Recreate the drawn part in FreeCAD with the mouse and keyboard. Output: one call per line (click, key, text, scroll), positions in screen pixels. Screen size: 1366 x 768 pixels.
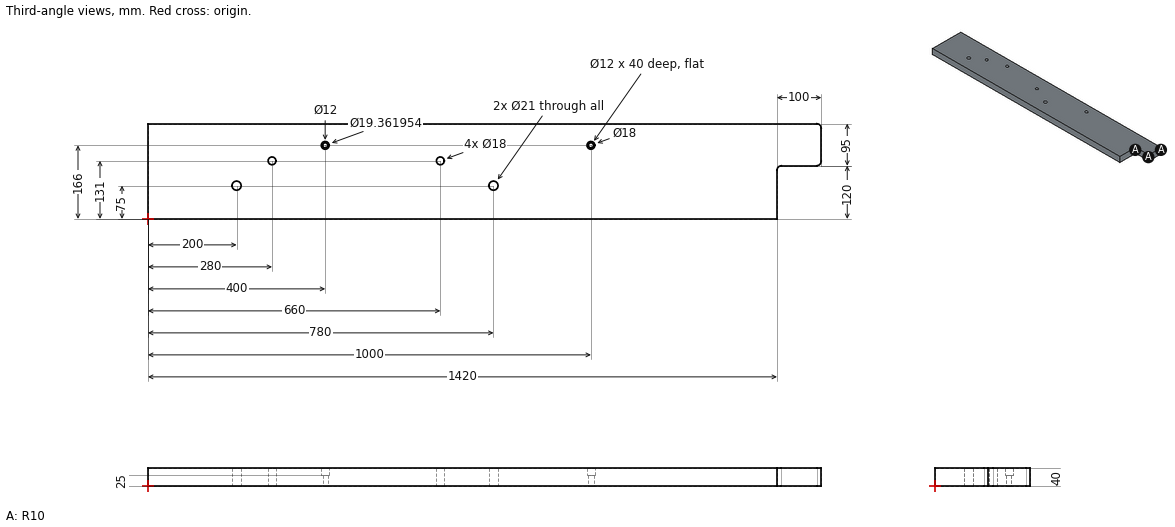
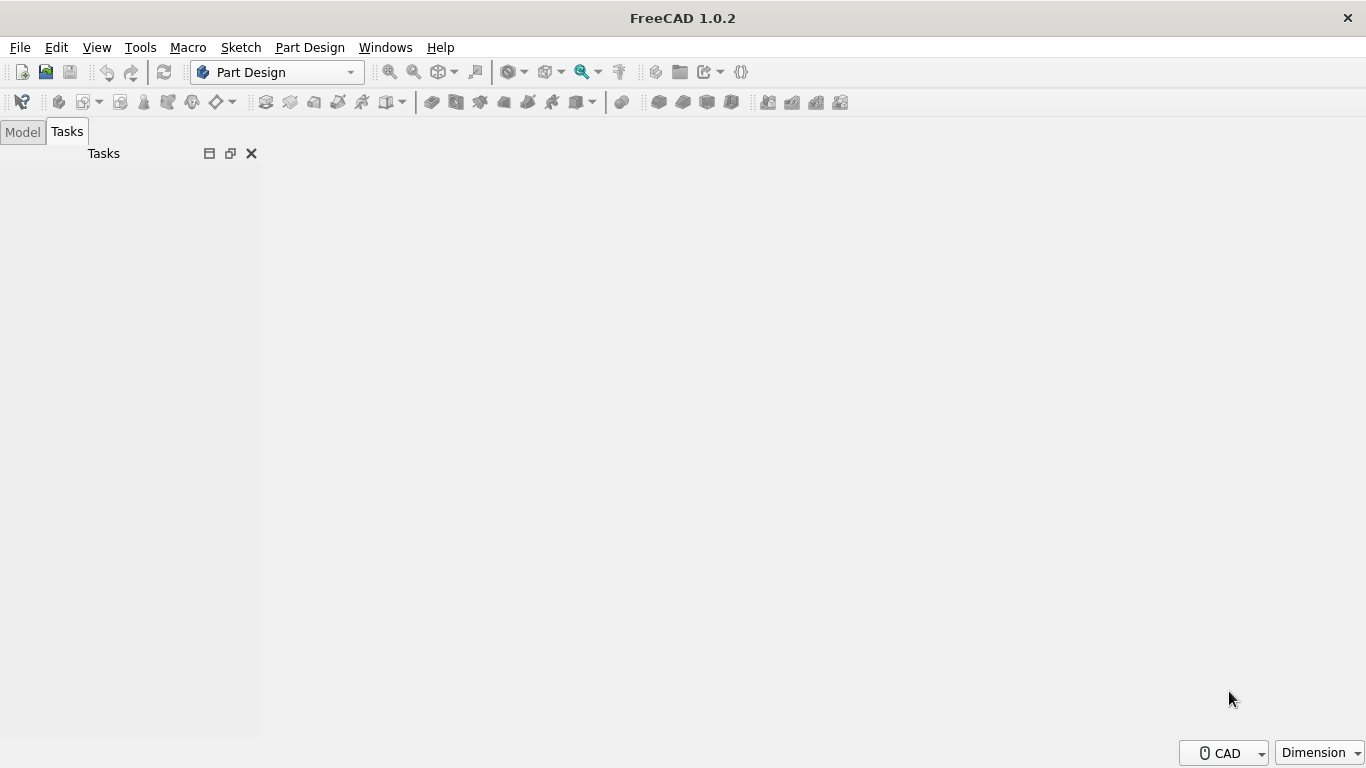
key(ctrl+n)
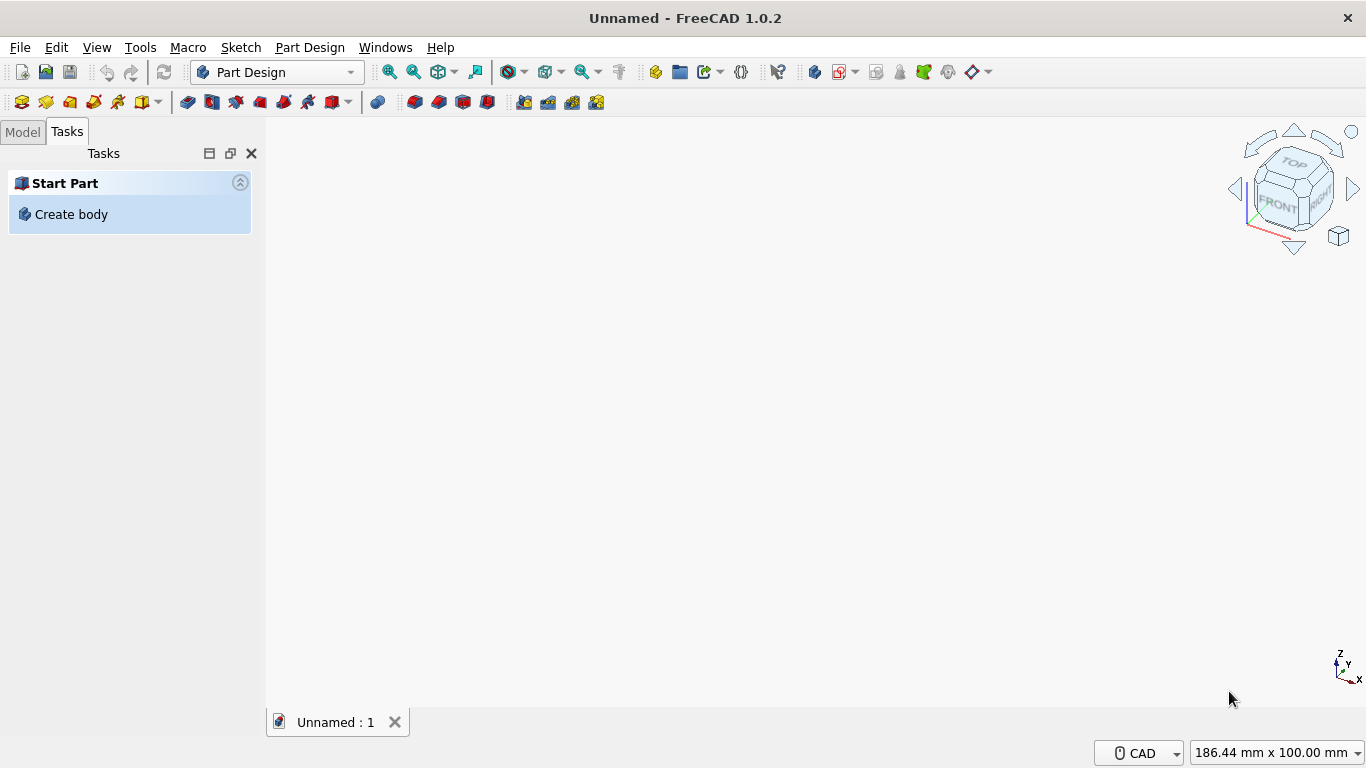
click(840, 72)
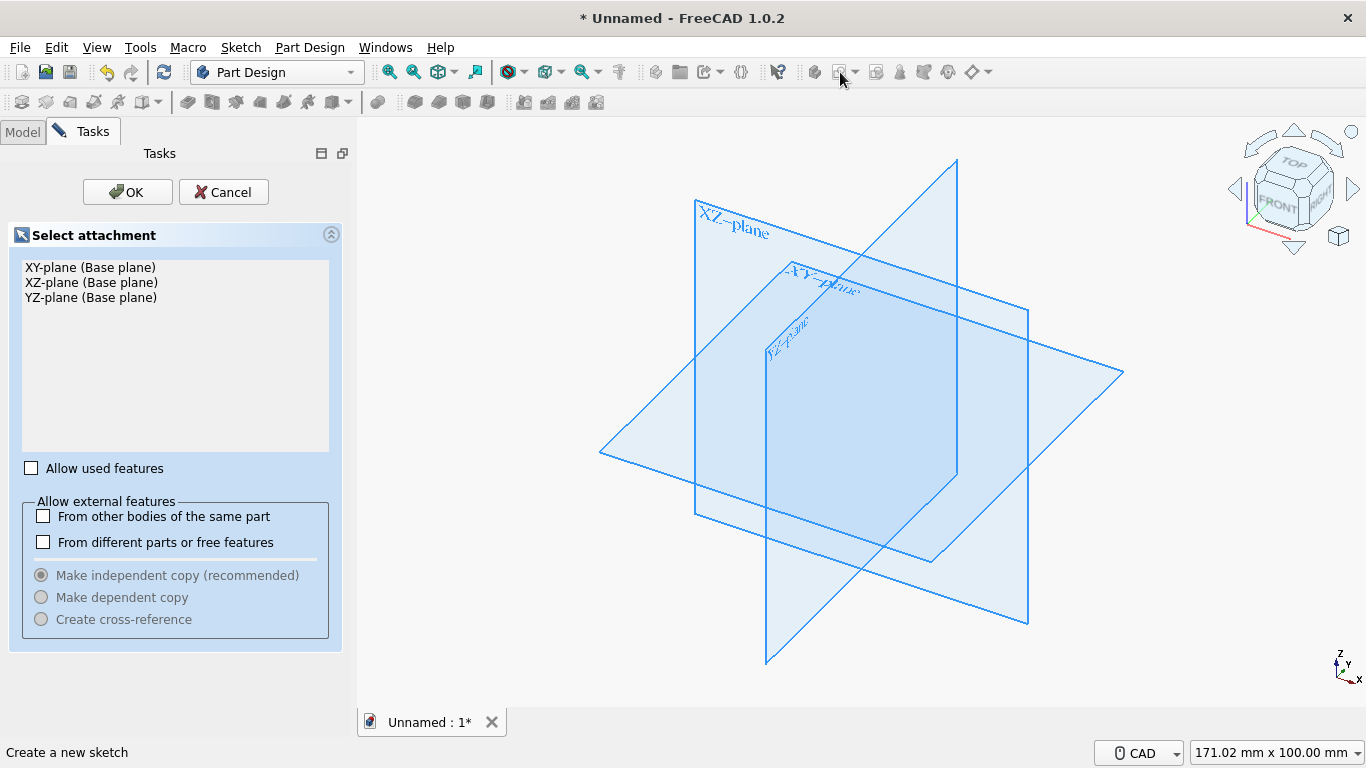
click(82, 268)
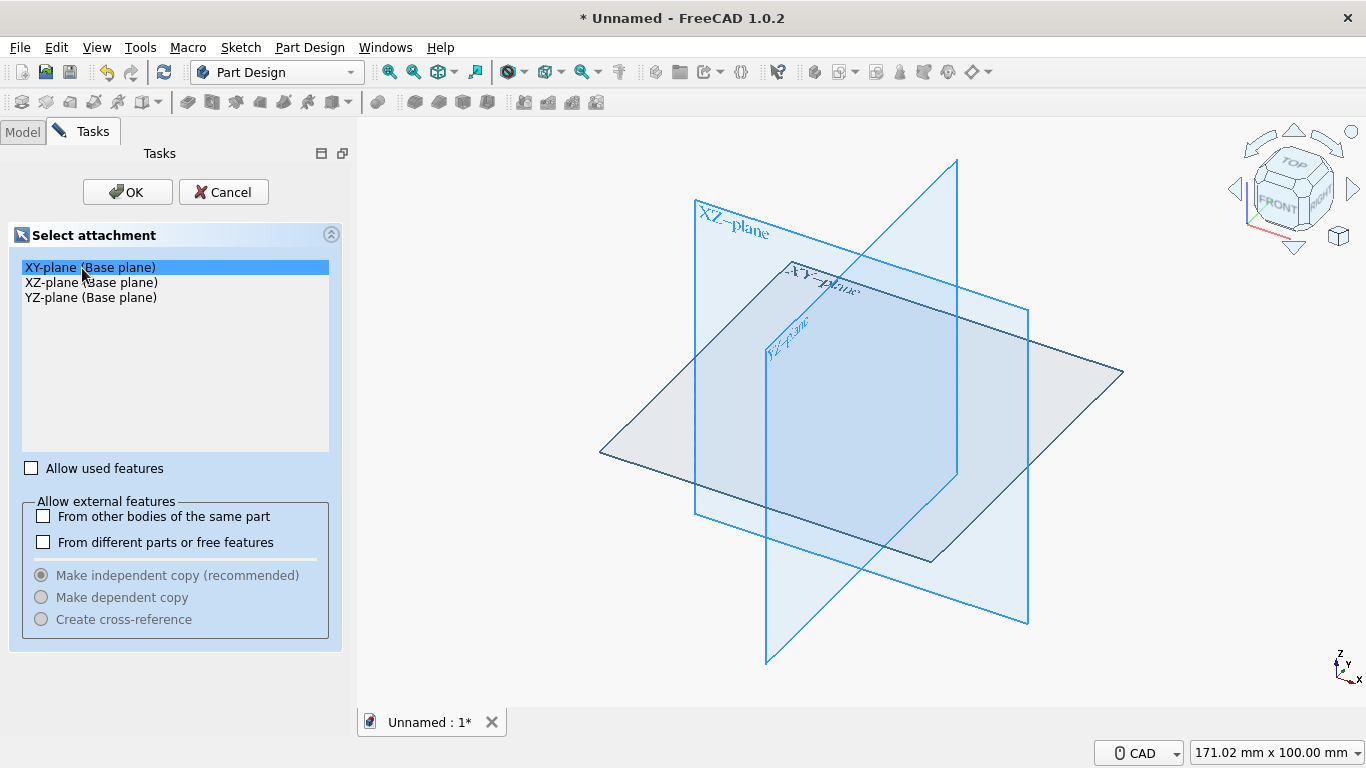
click(128, 192)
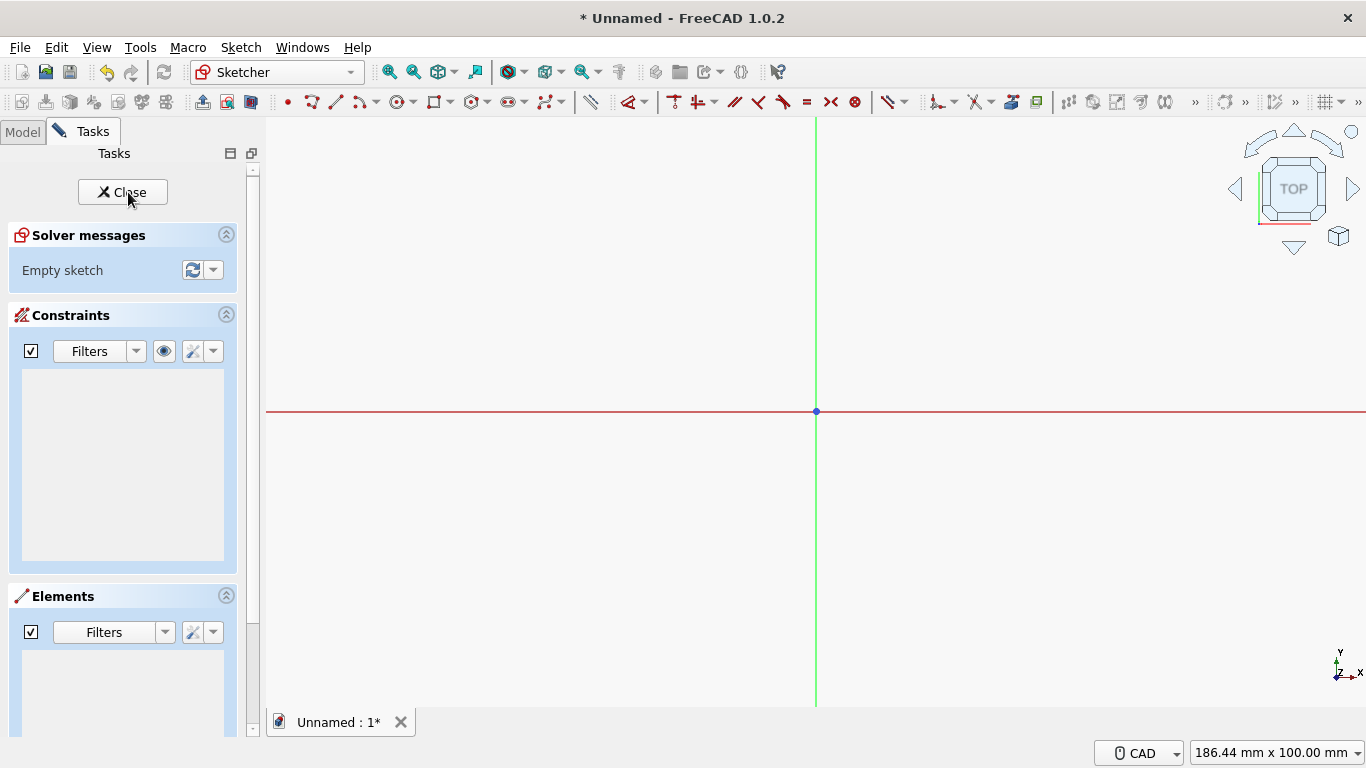
scroll(382, 463, down, 13)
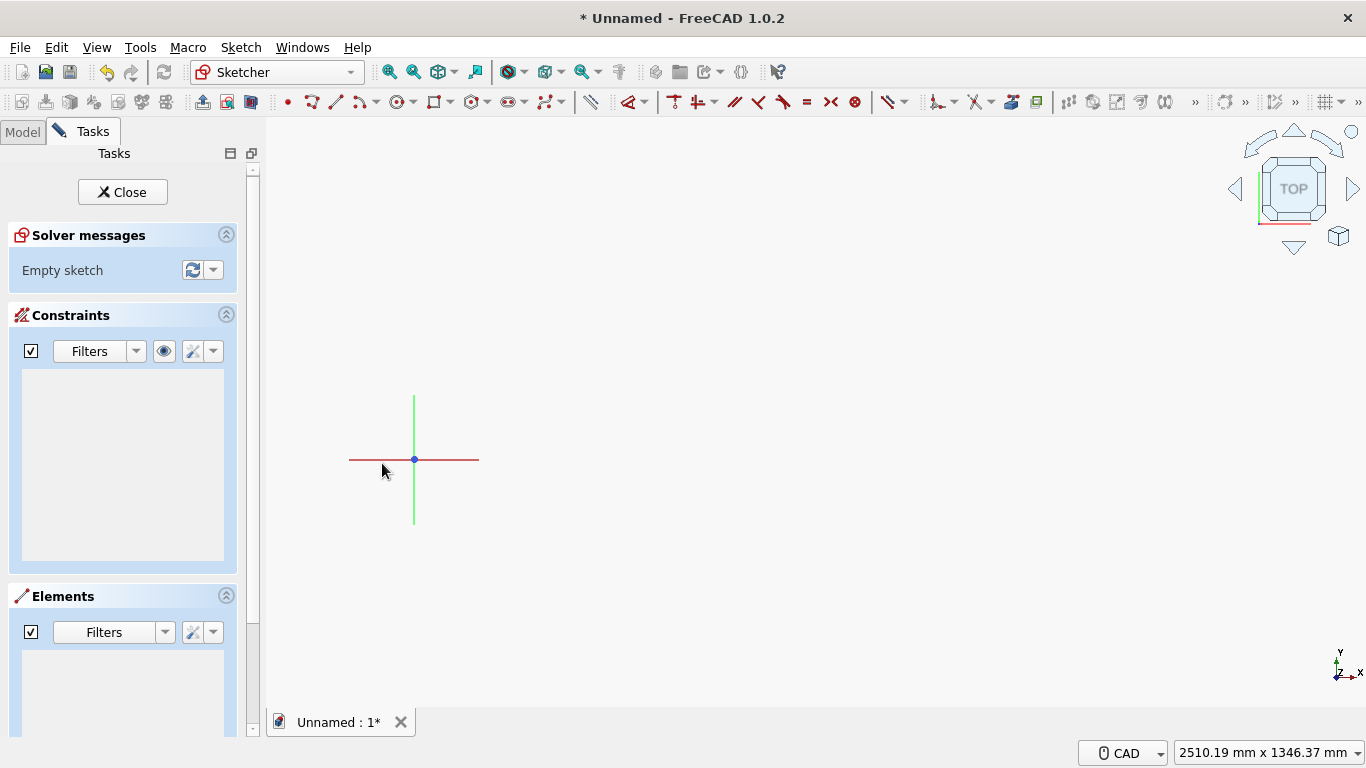
key(g)
key(m)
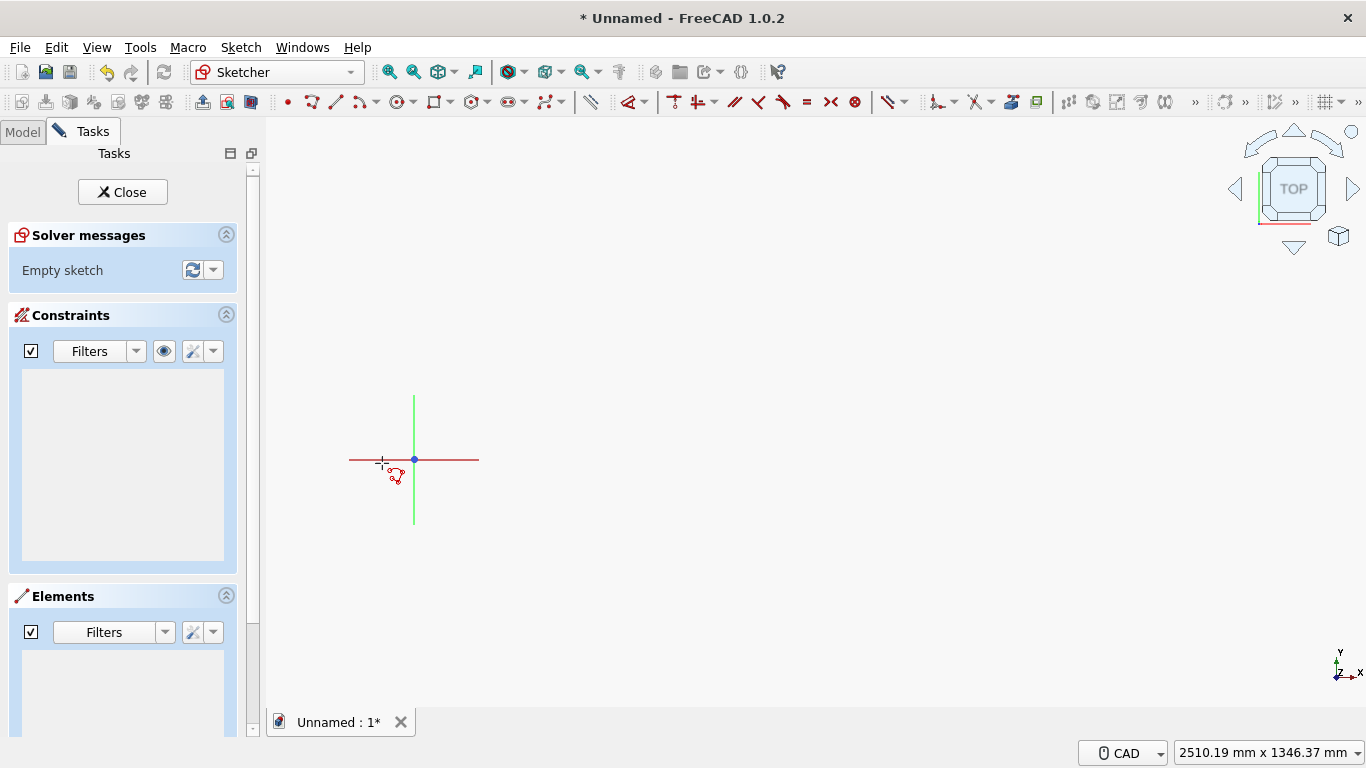
click(414, 460)
click(1037, 451)
click(1037, 407)
click(1080, 407)
click(1080, 366)
click(423, 366)
click(414, 460)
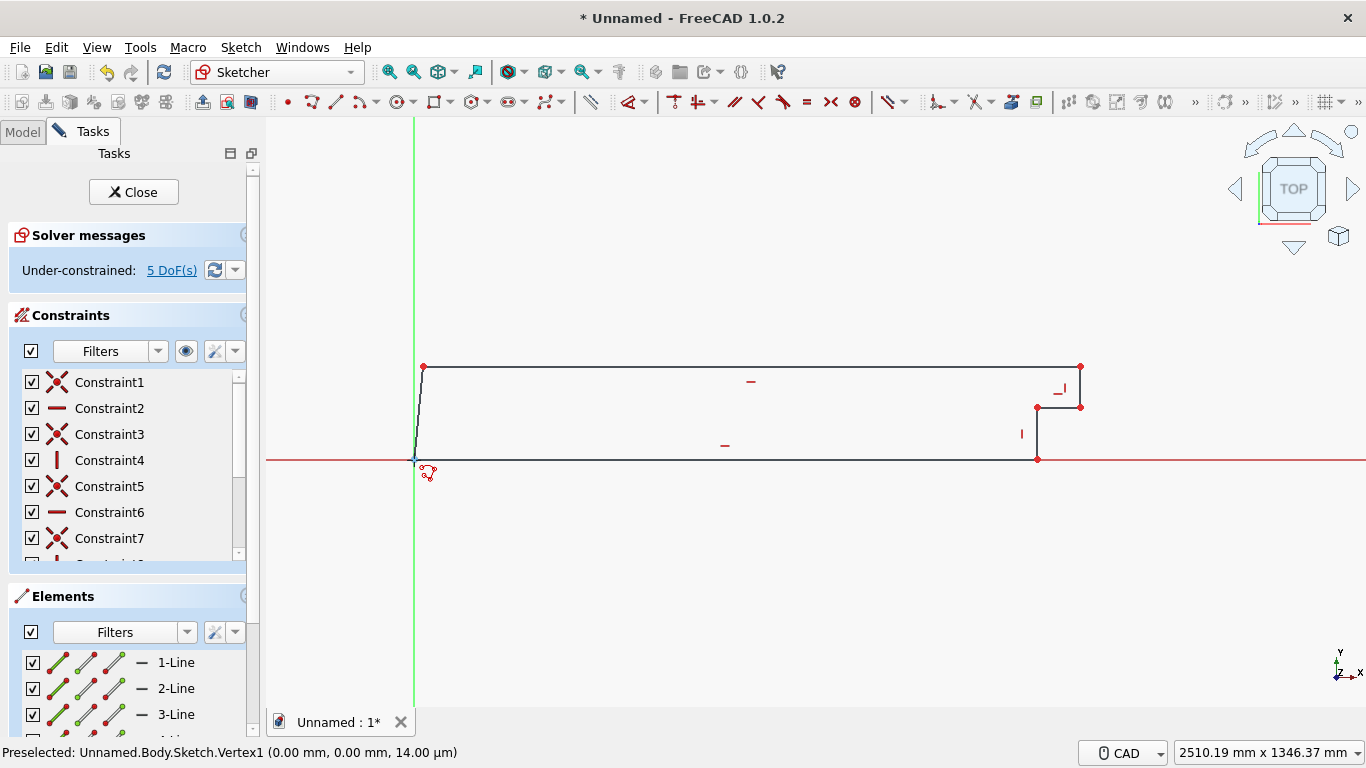
key(g)
key(c)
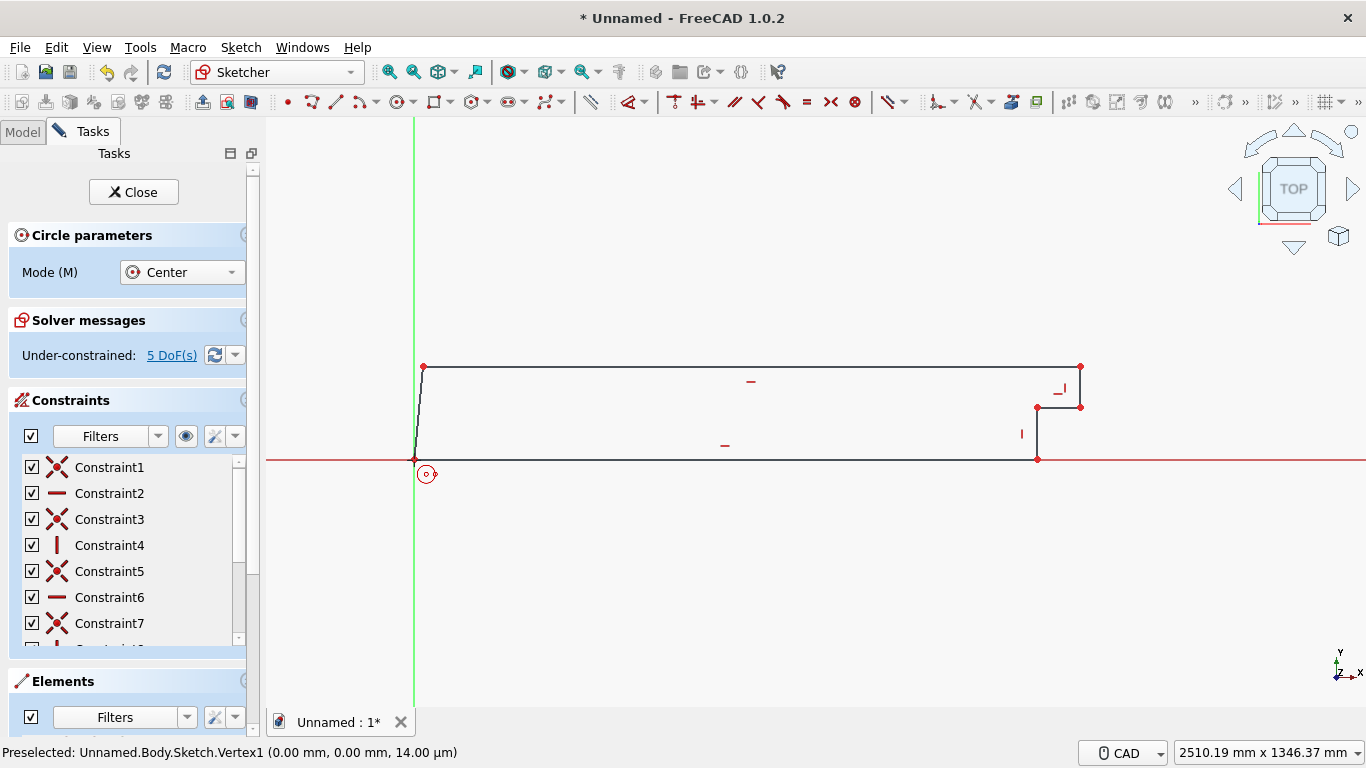
scroll(704, 402, up, 9)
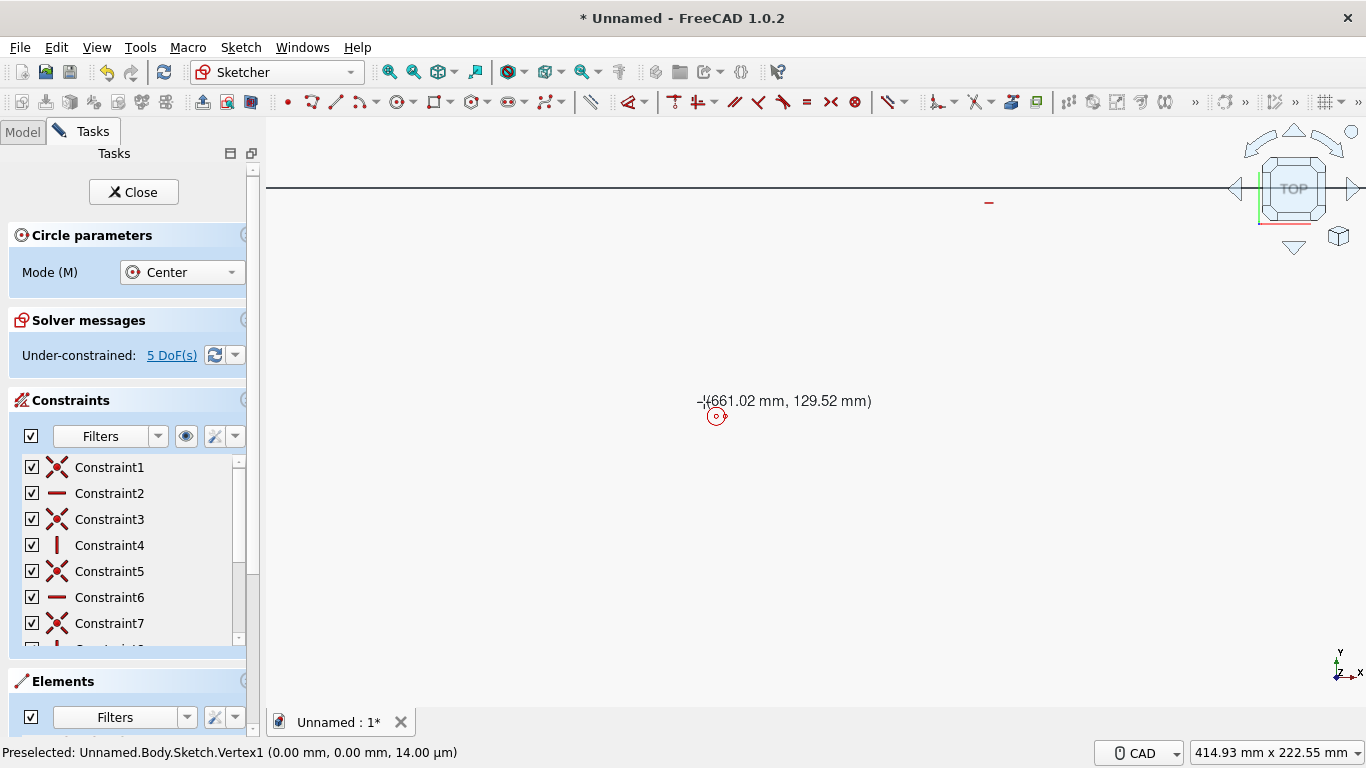
scroll(705, 402, down, 9)